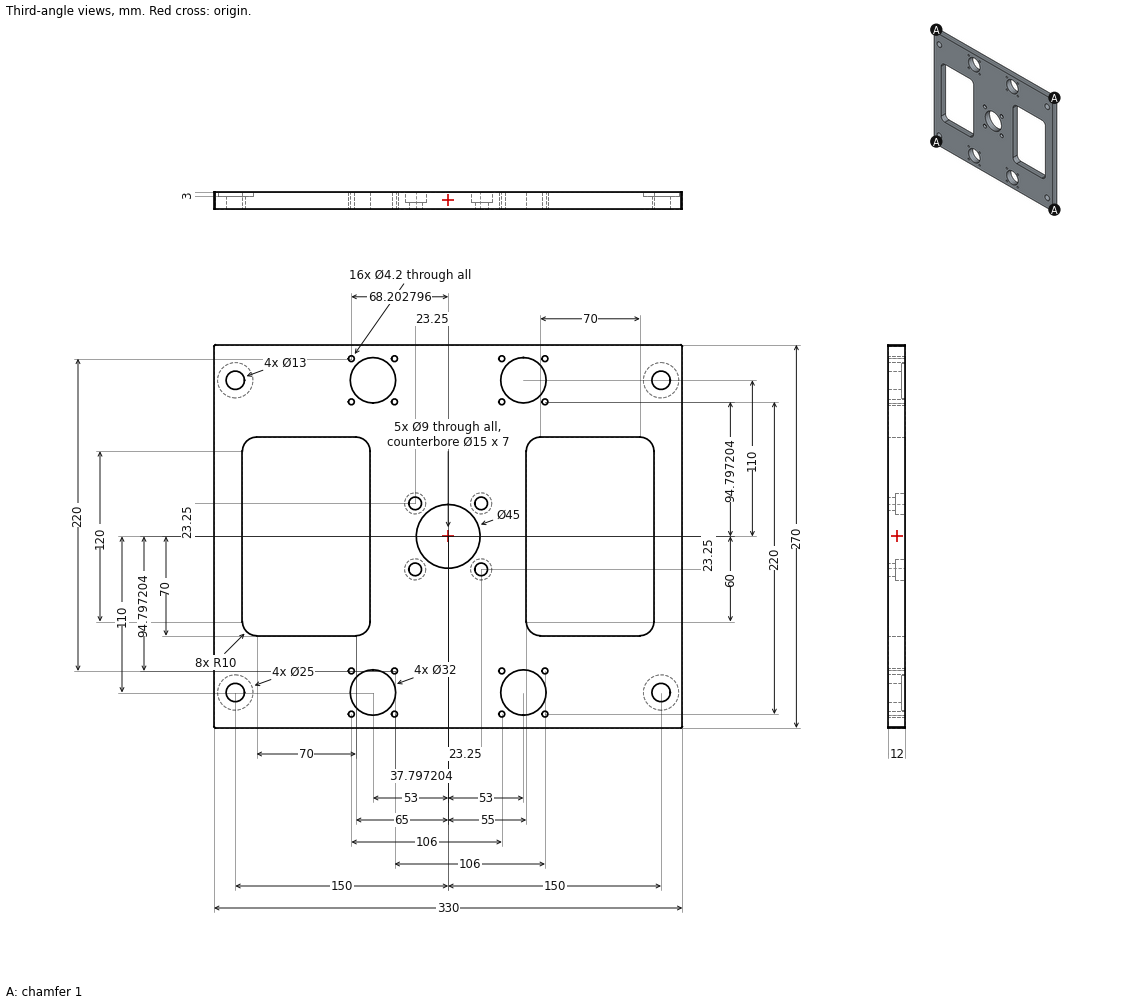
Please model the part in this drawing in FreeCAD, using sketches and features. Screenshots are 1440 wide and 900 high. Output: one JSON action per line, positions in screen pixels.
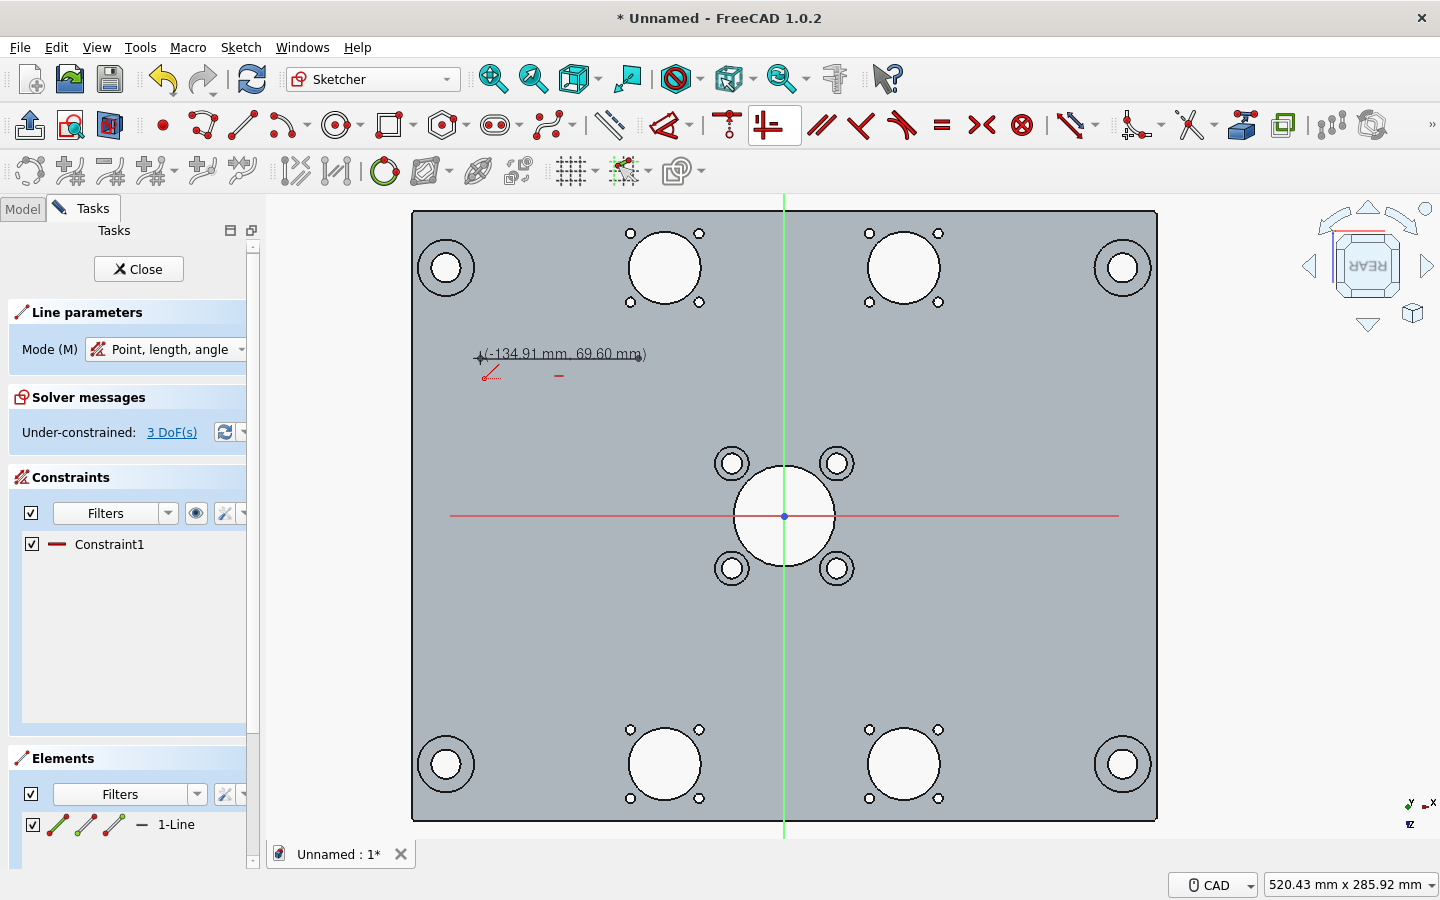
{"action": "left_click", "coordinate": [457, 381]}
{"action": "left_click", "coordinate": [457, 651]}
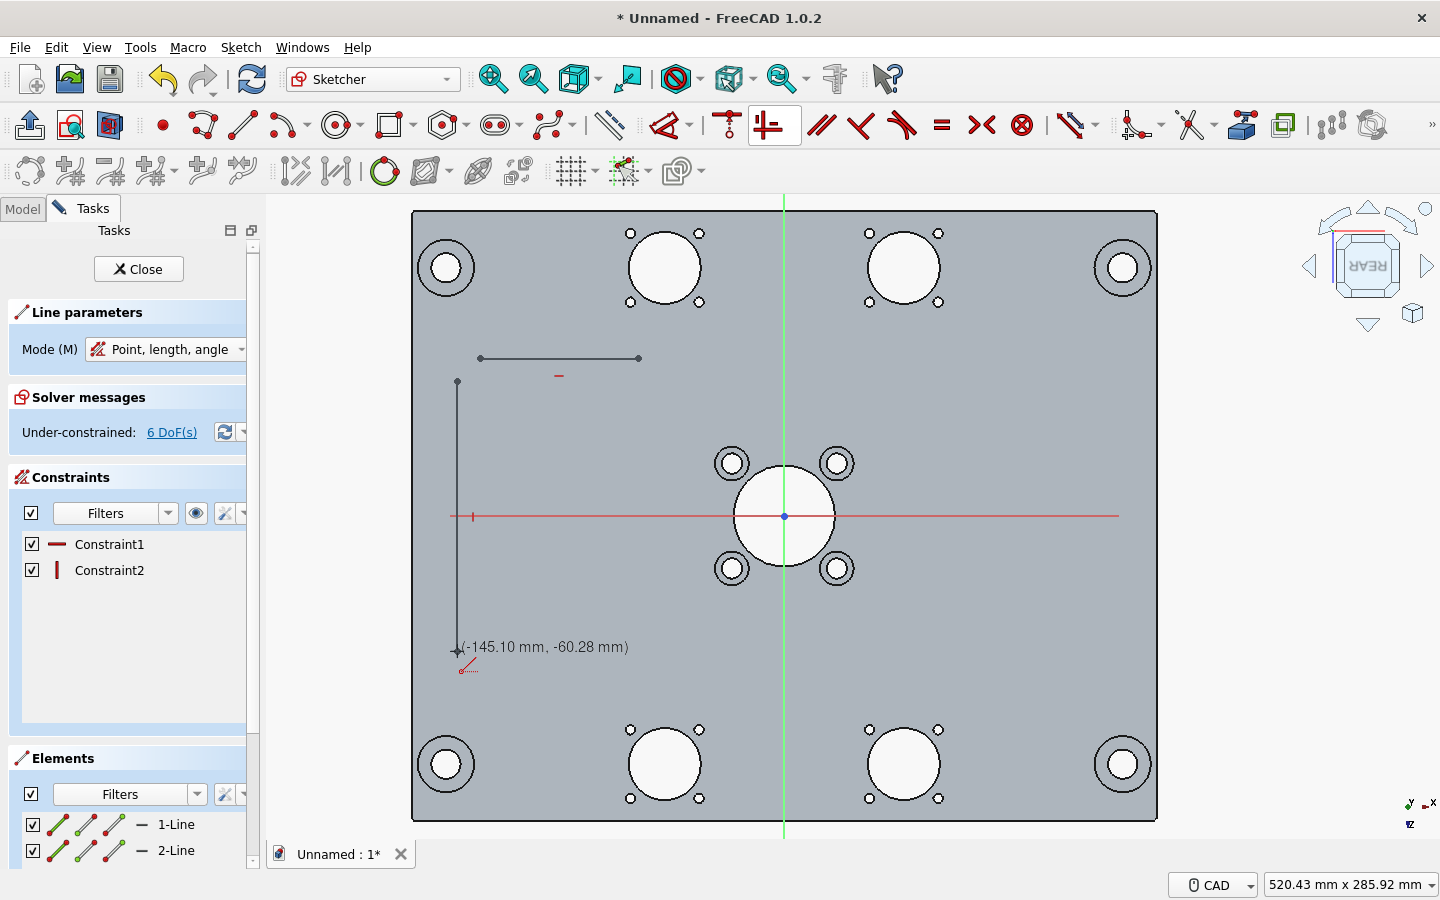
{"action": "left_click", "coordinate": [480, 674]}
{"action": "left_click", "coordinate": [638, 674]}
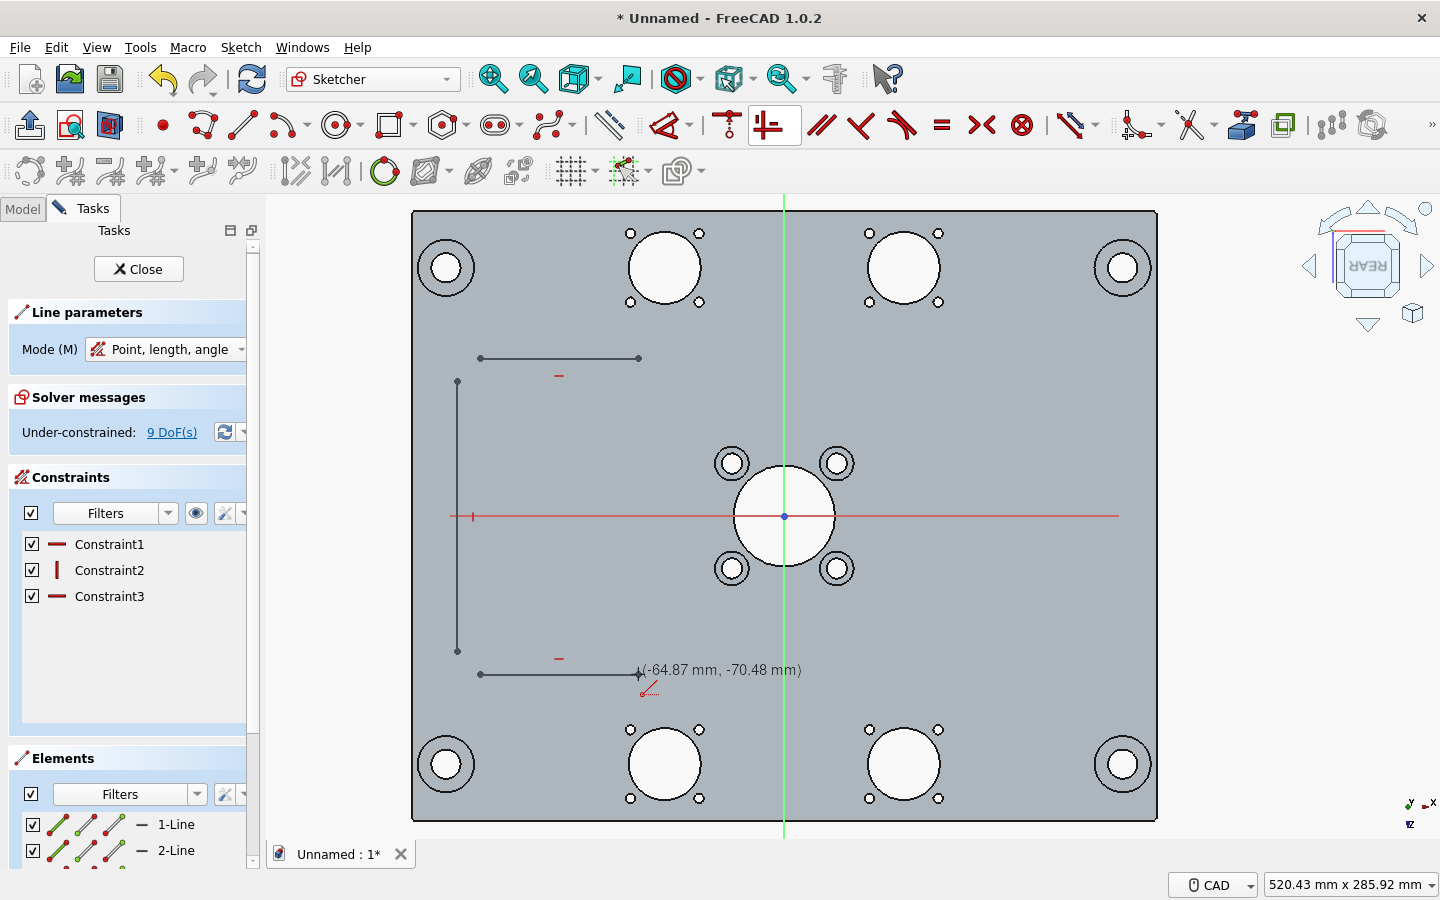
{"action": "left_click", "coordinate": [660, 651]}
{"action": "left_click", "coordinate": [660, 381]}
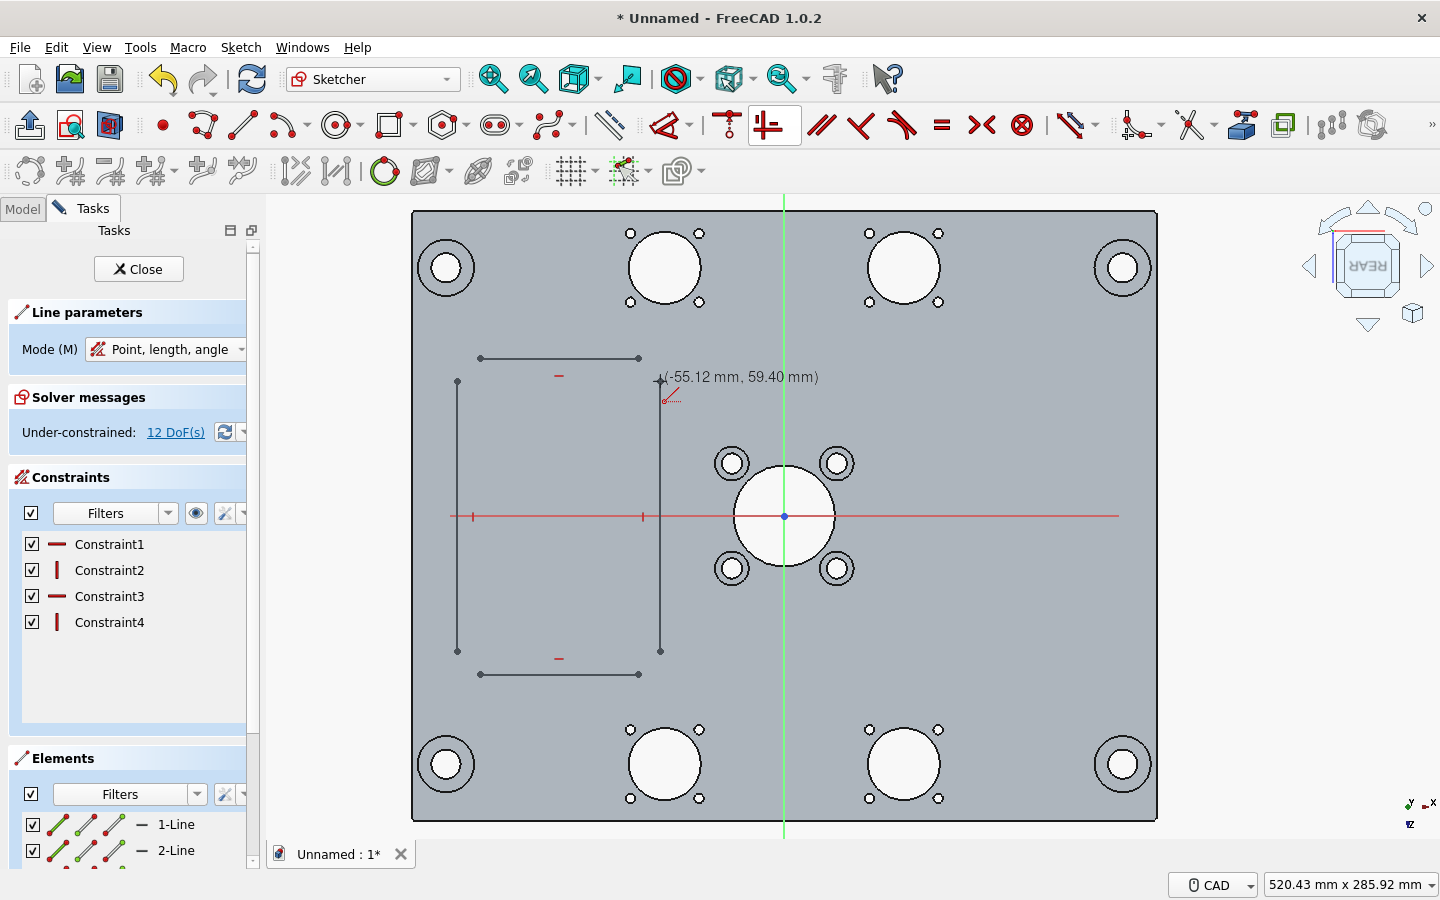
{"action": "key", "text": "g 3 a"}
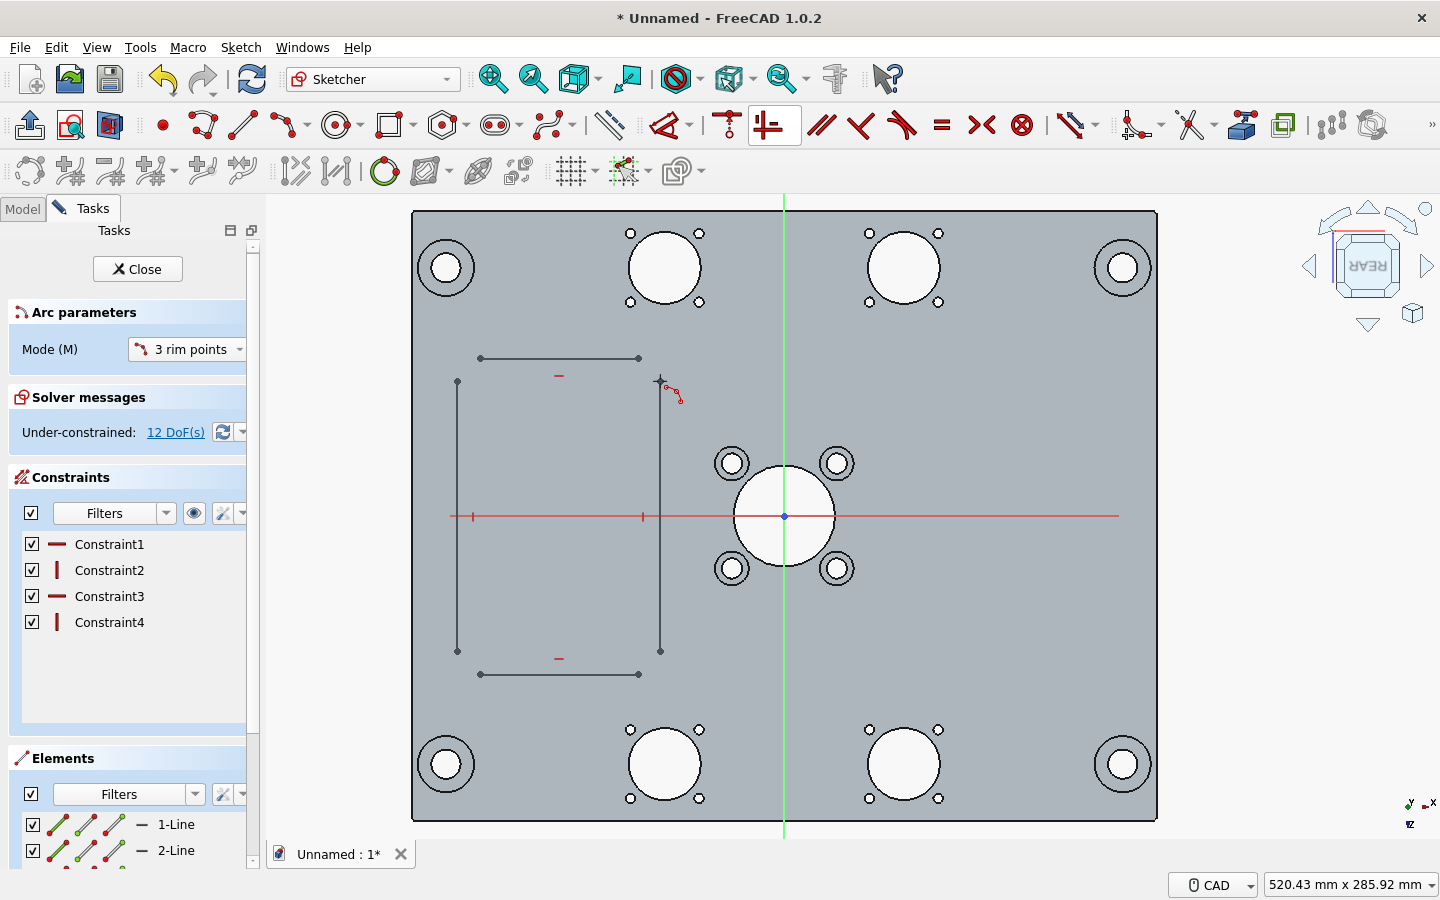
{"action": "left_click", "coordinate": [480, 359]}
{"action": "left_click", "coordinate": [457, 382]}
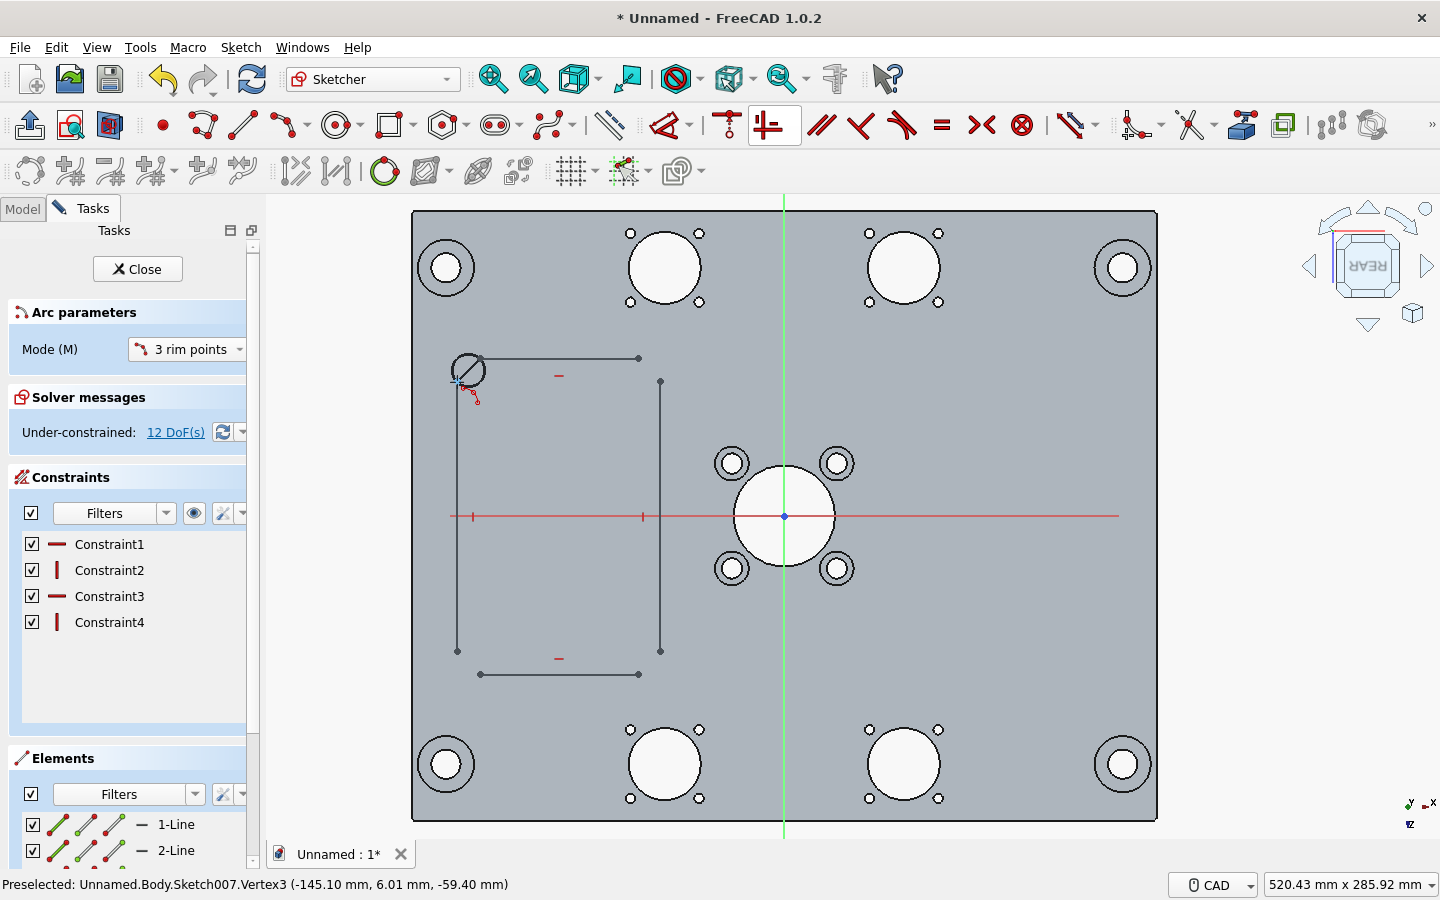
{"action": "scroll", "coordinate": [464, 365], "scroll_direction": "up", "scroll_amount": 5}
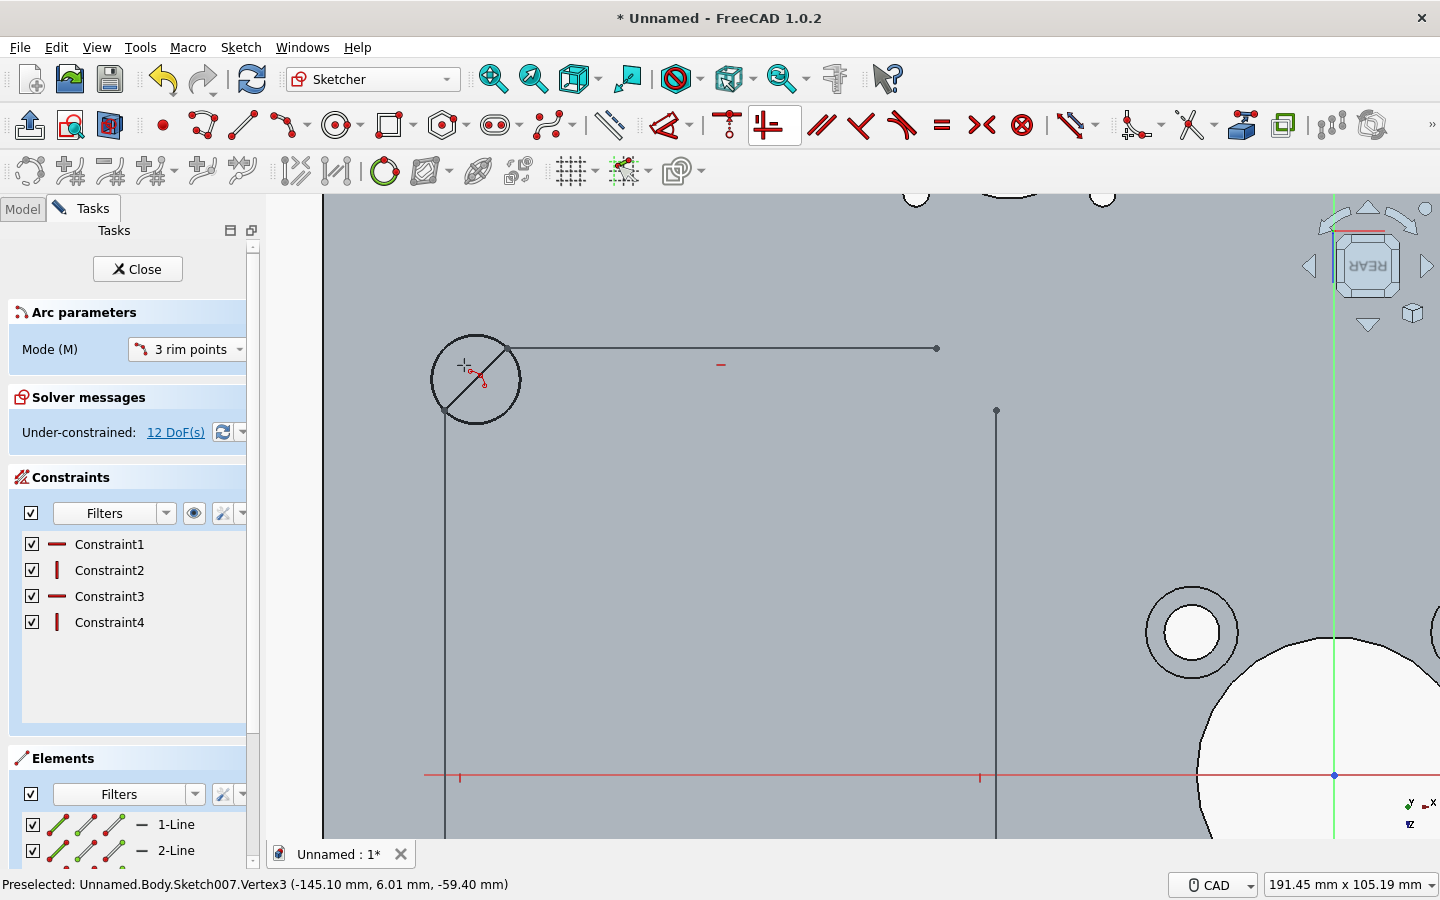
{"action": "left_click", "coordinate": [463, 364]}